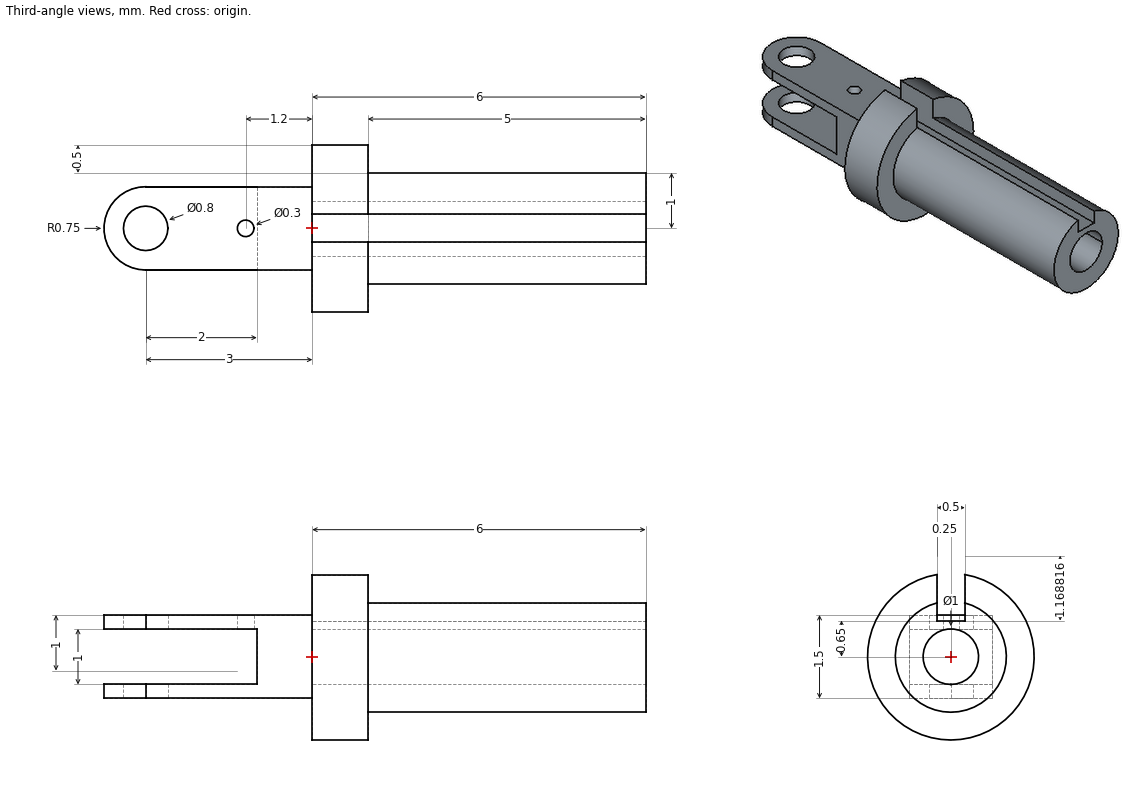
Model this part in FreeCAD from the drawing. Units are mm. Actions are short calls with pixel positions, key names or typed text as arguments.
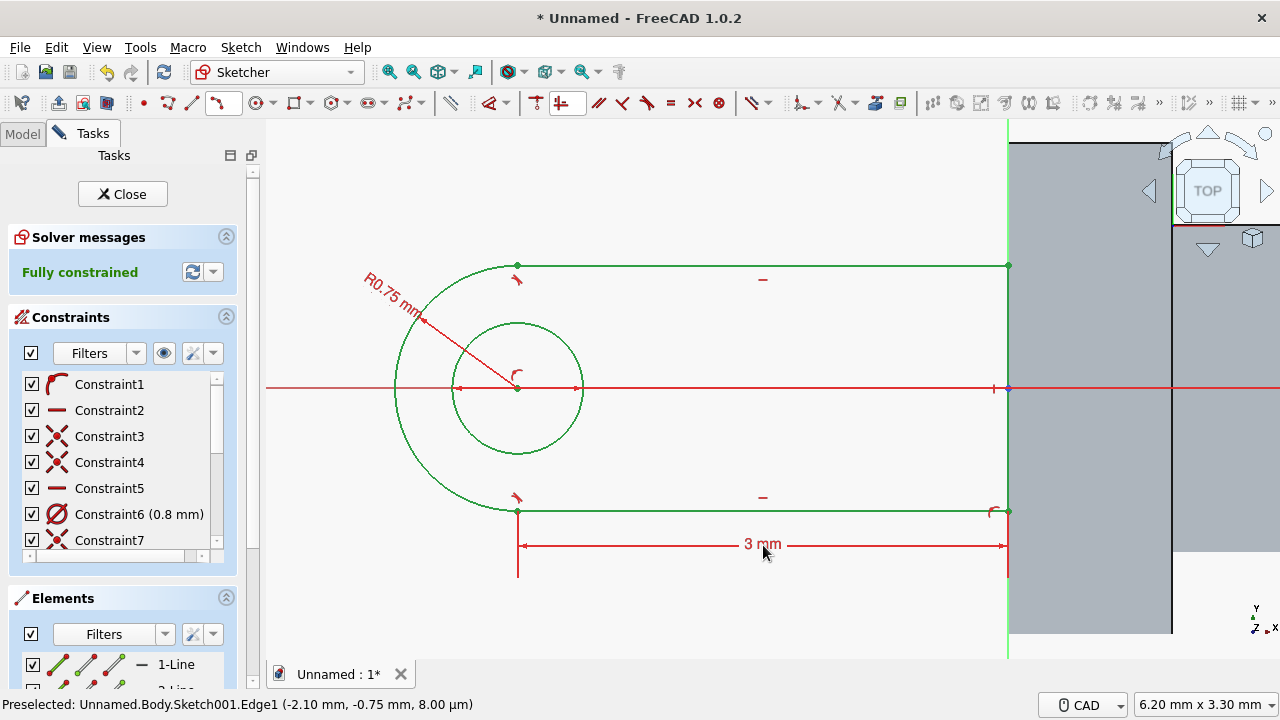
click(123, 194)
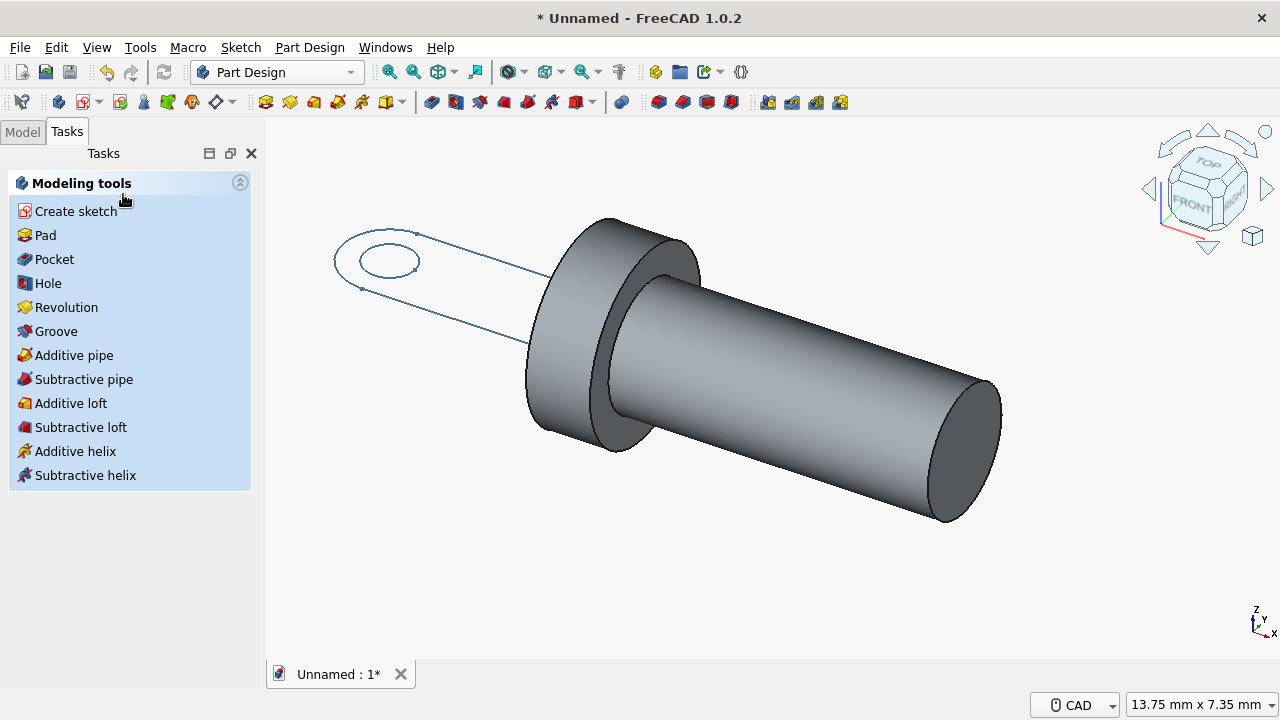
click(266, 102)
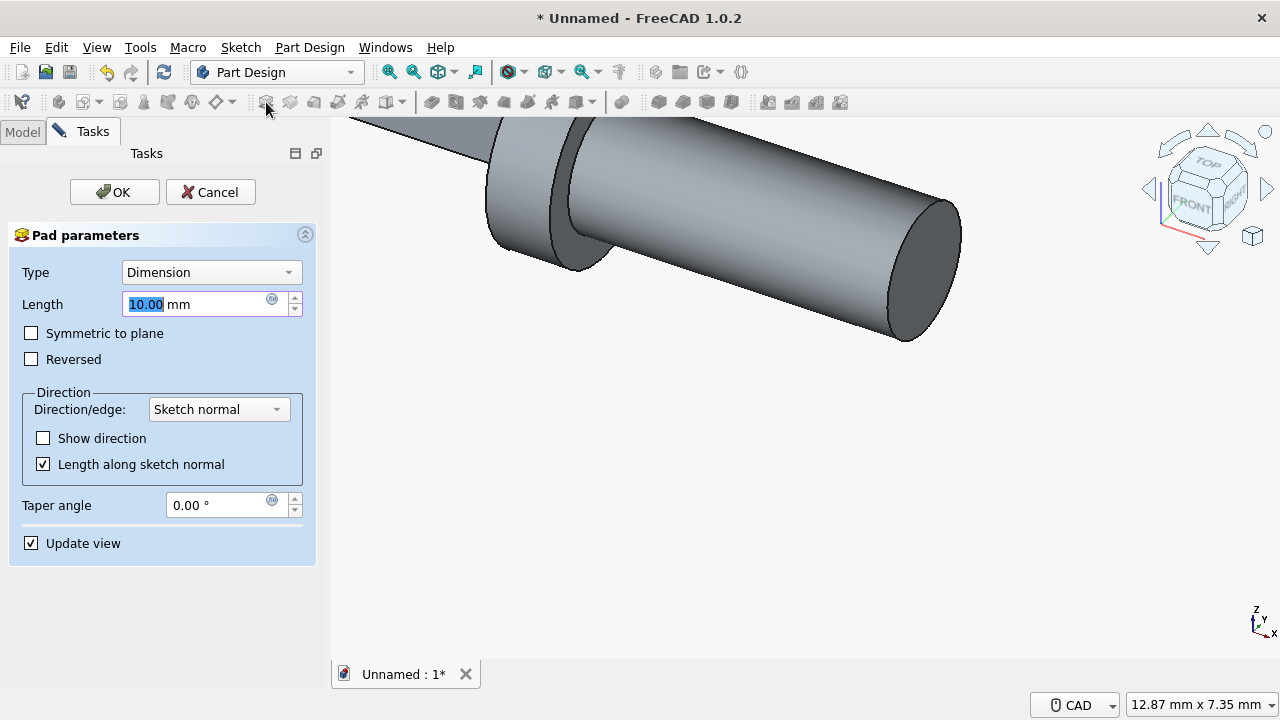
text(1.5)
key(Tab)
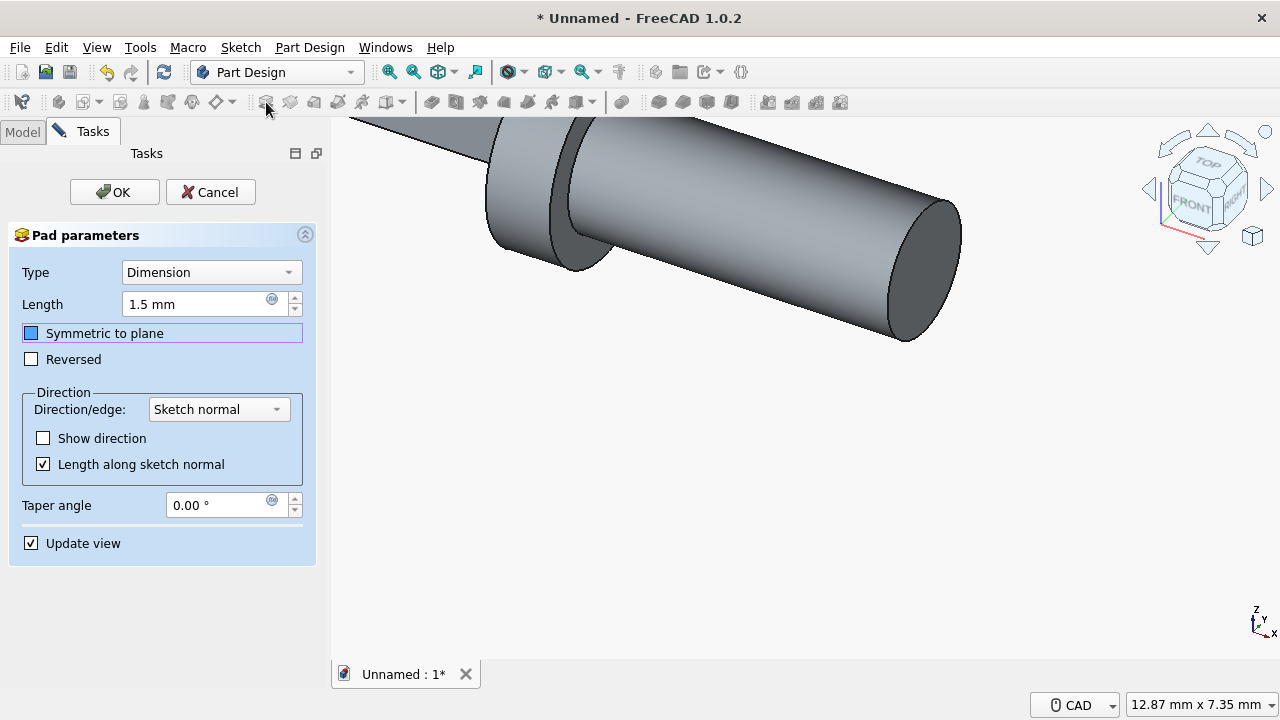
click(30, 333)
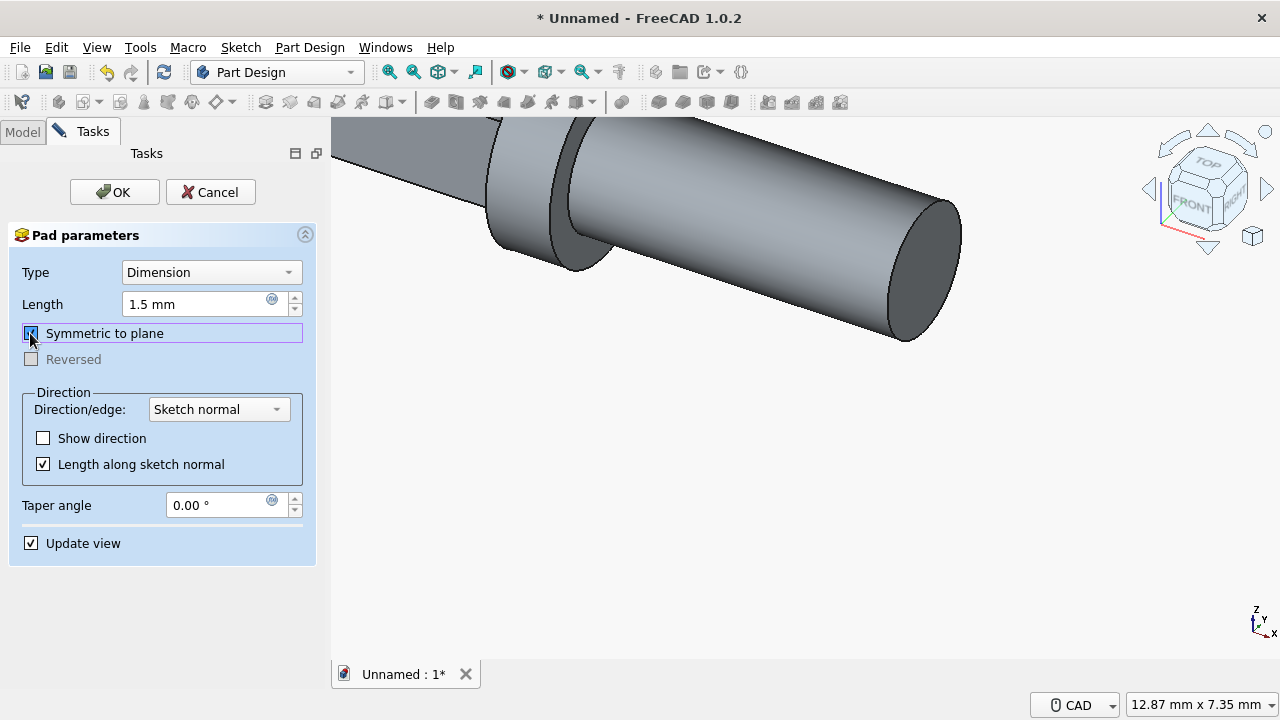
click(115, 192)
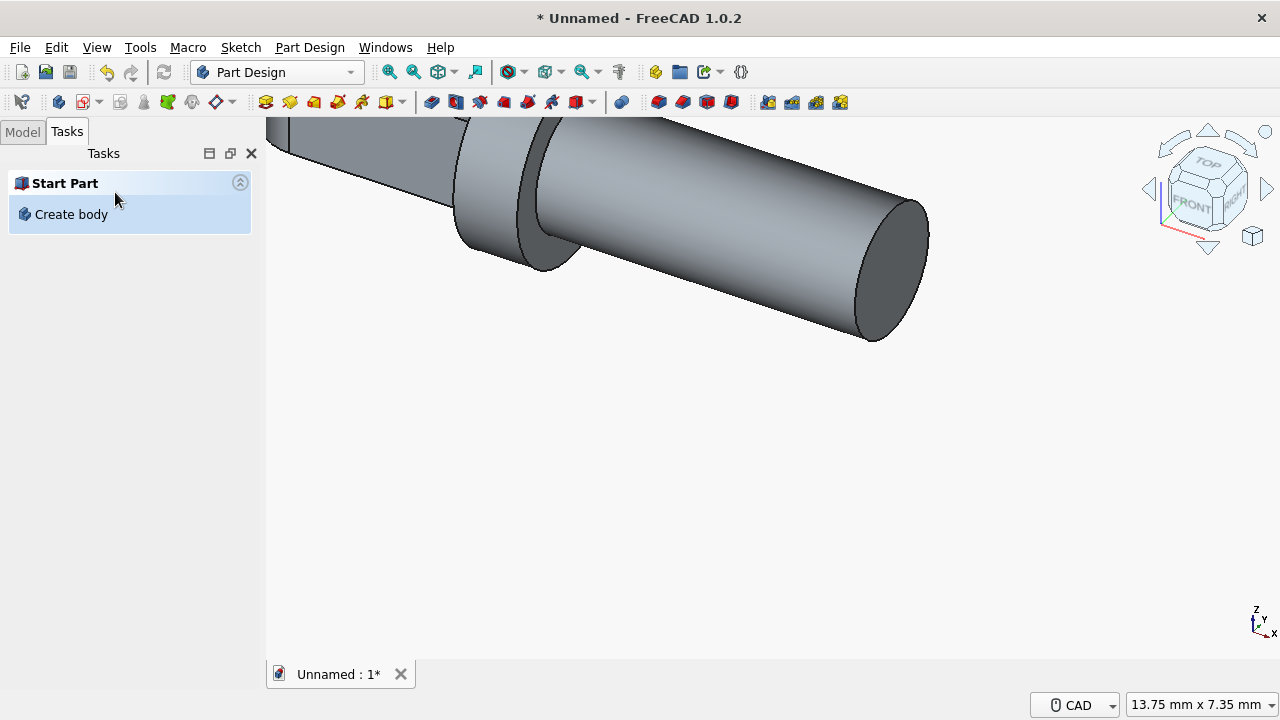
click(390, 72)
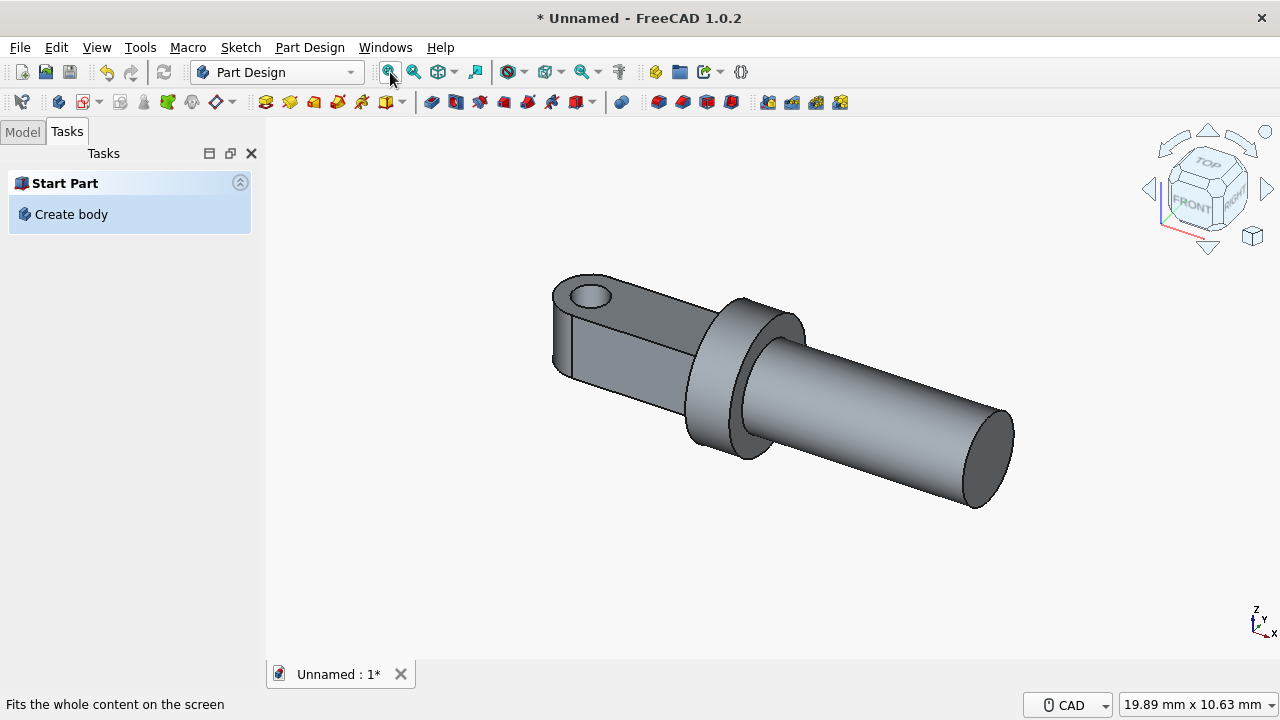
click(84, 102)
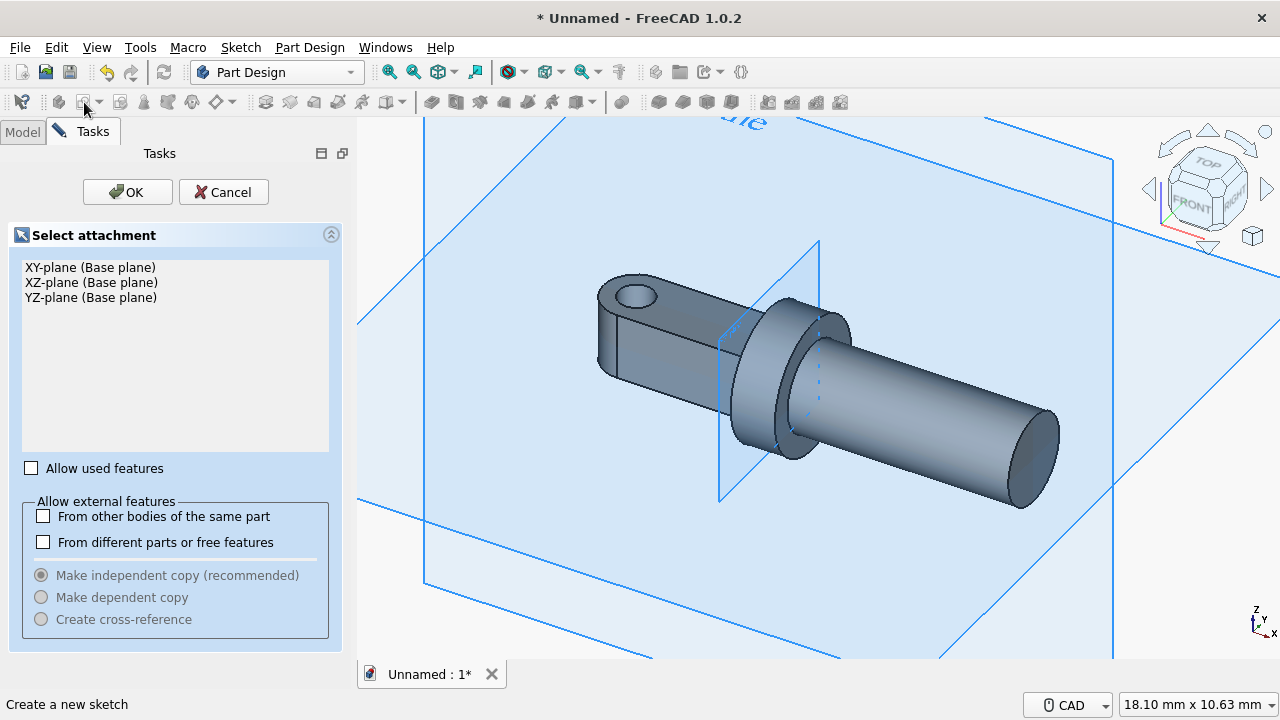
click(82, 268)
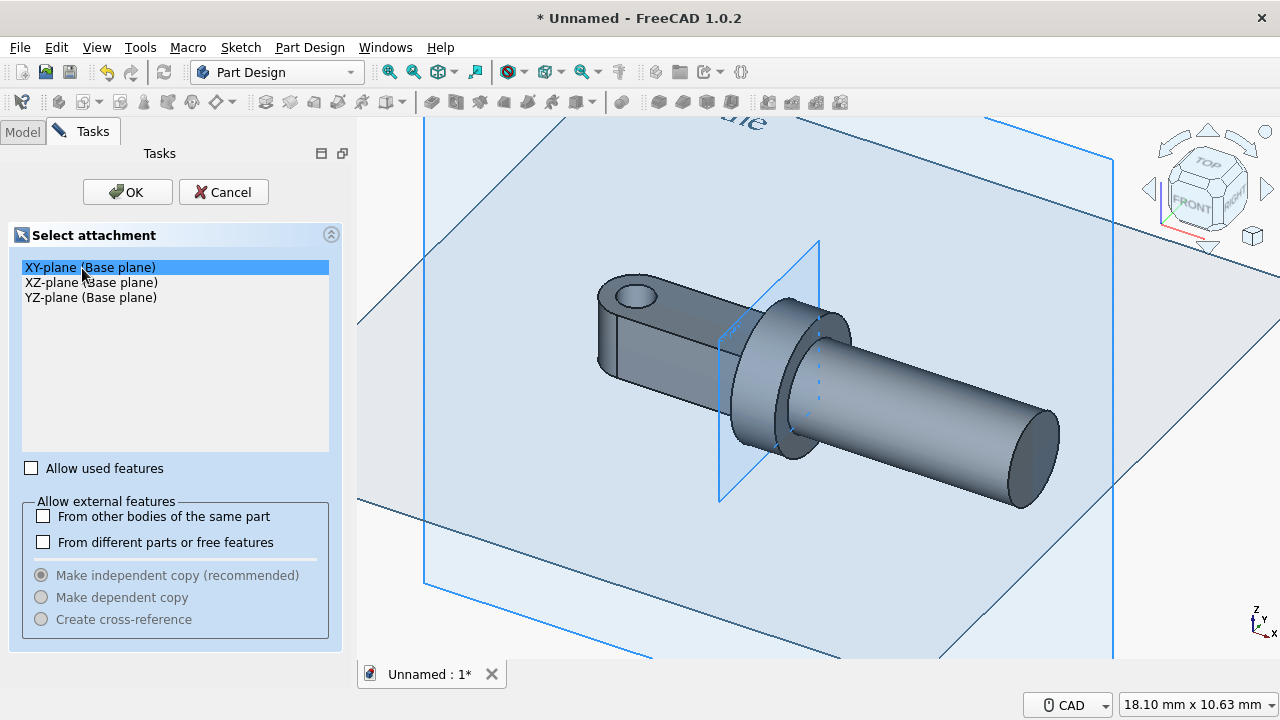
click(128, 192)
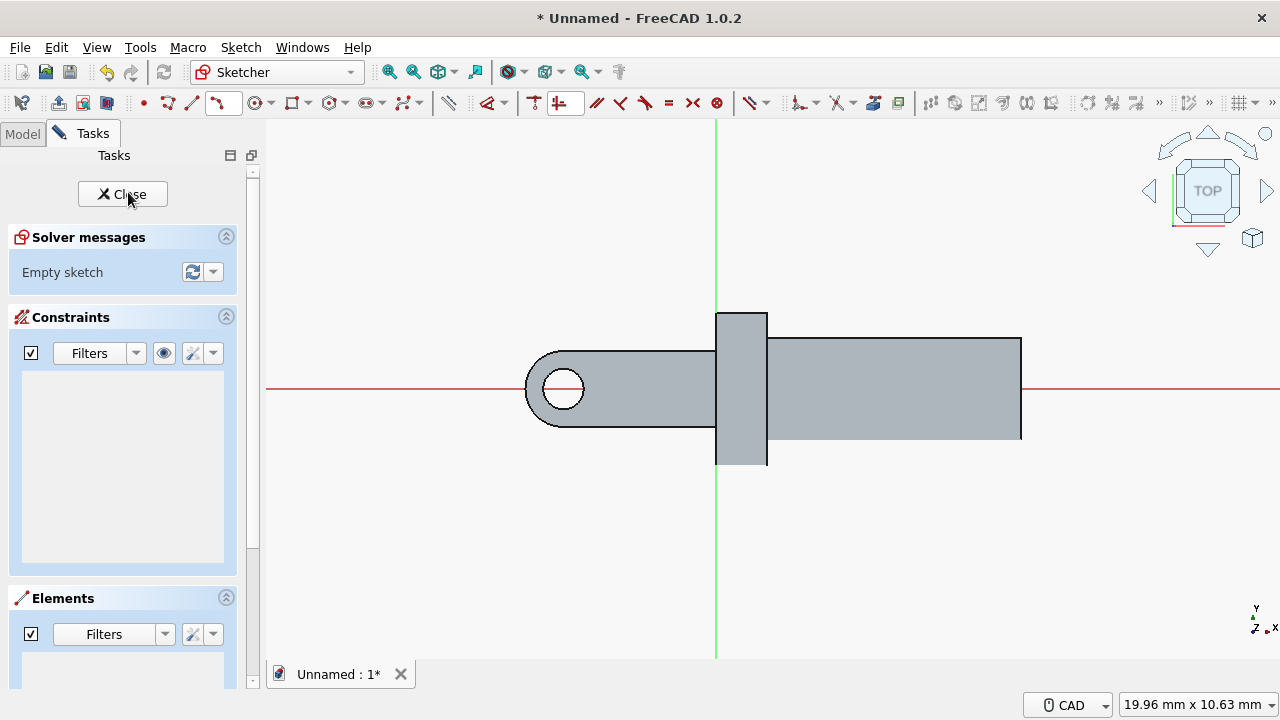
click(108, 104)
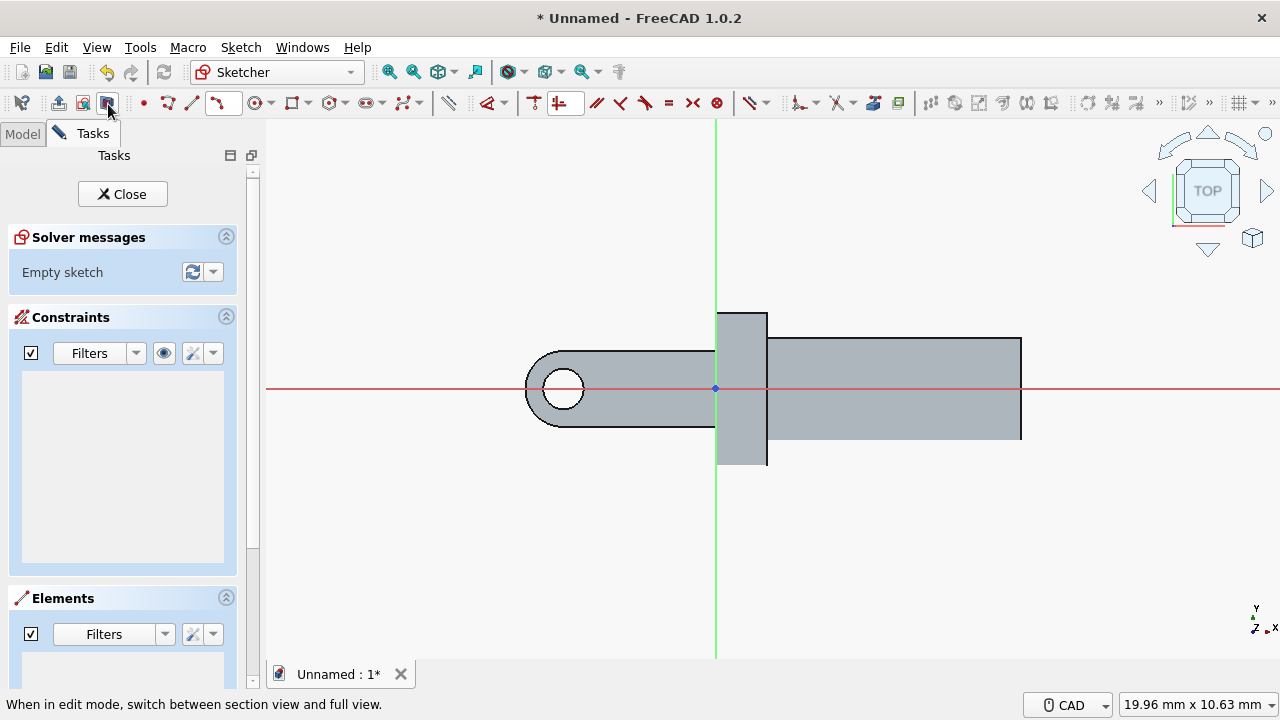
scroll(584, 389, up, 6)